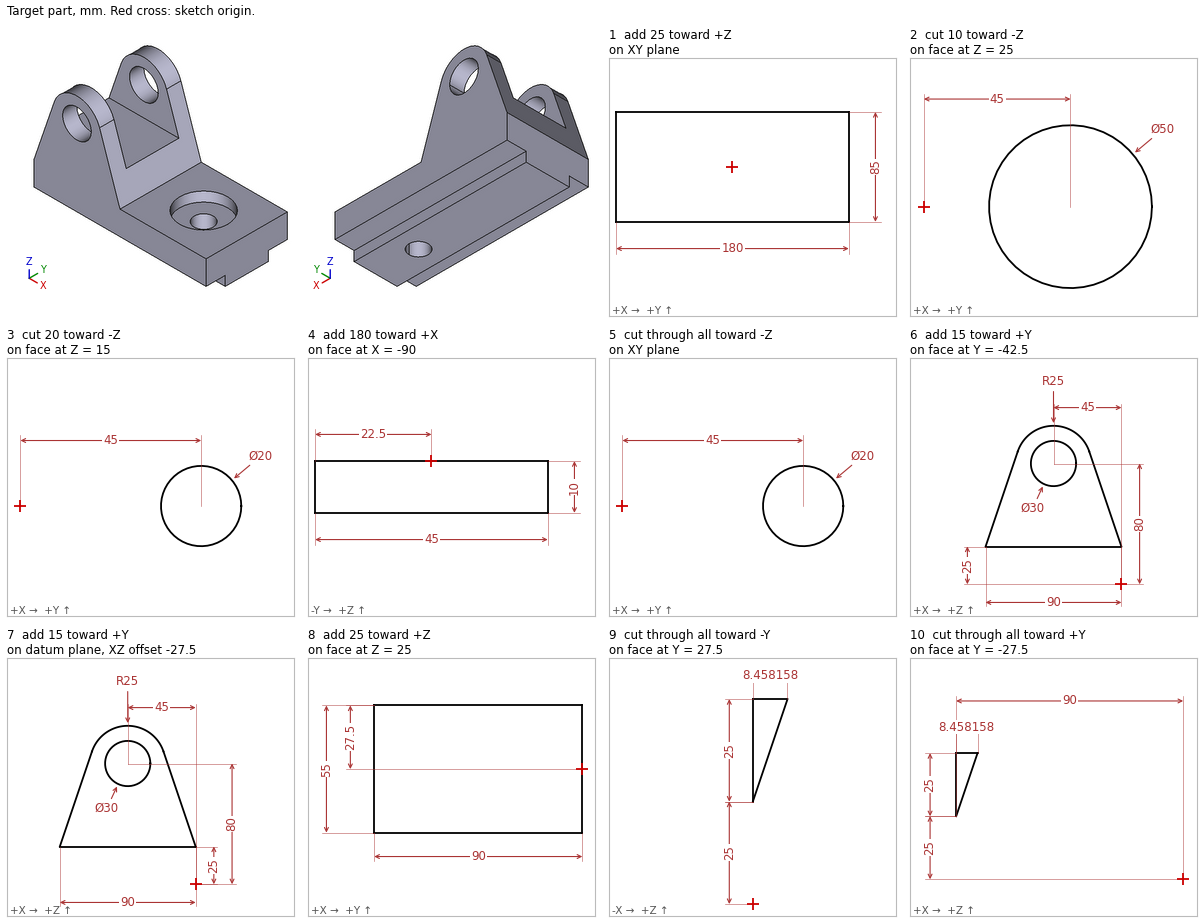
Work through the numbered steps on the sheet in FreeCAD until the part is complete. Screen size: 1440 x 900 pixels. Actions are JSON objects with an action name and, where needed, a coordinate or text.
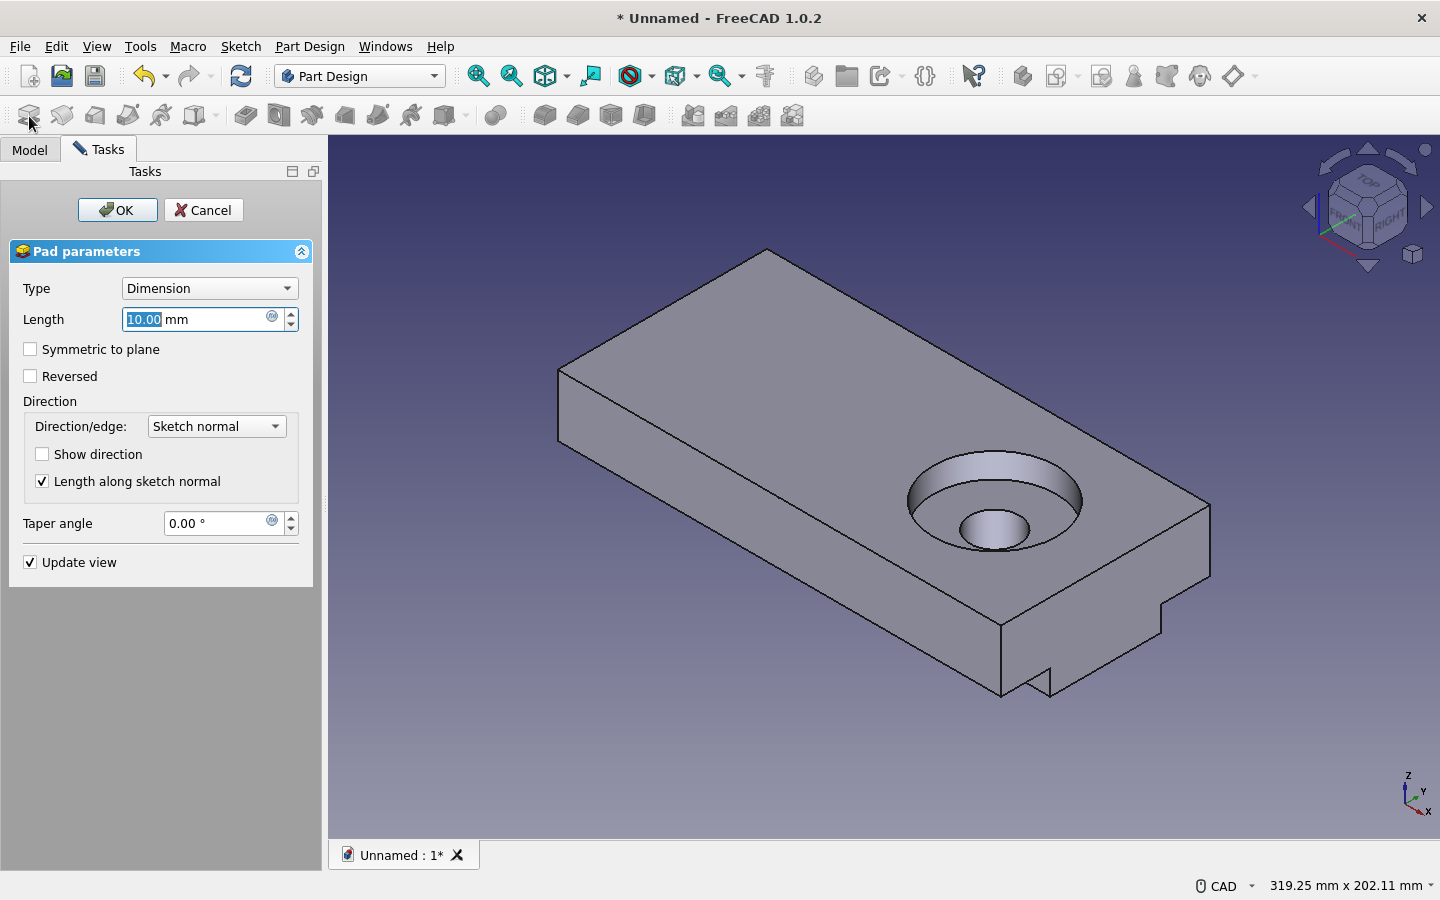
{"action": "type", "text": "15"}
{"action": "key", "text": "Tab"}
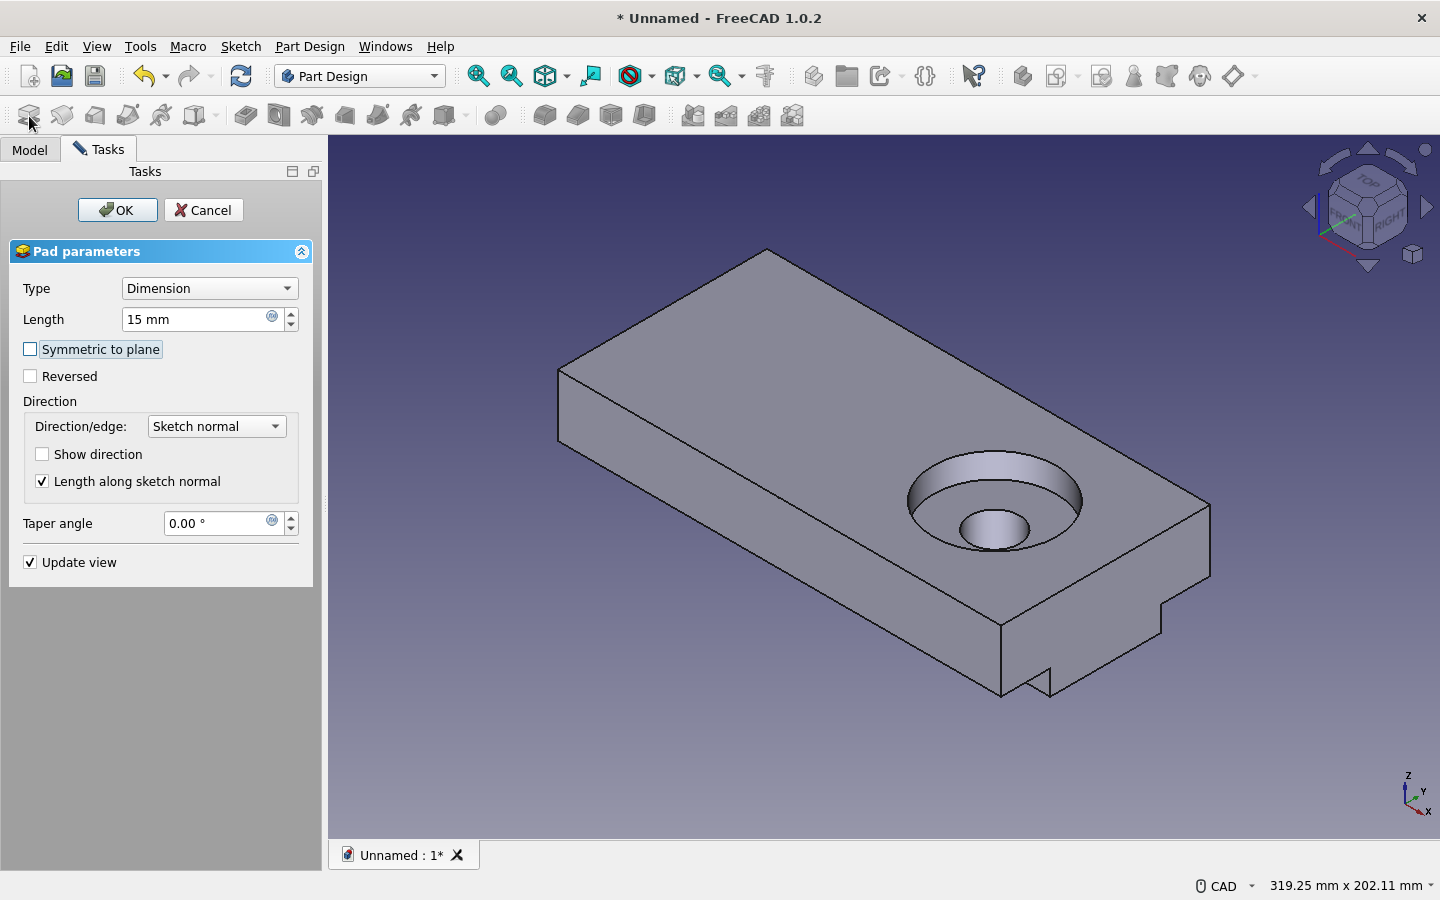
{"action": "left_click", "coordinate": [31, 376]}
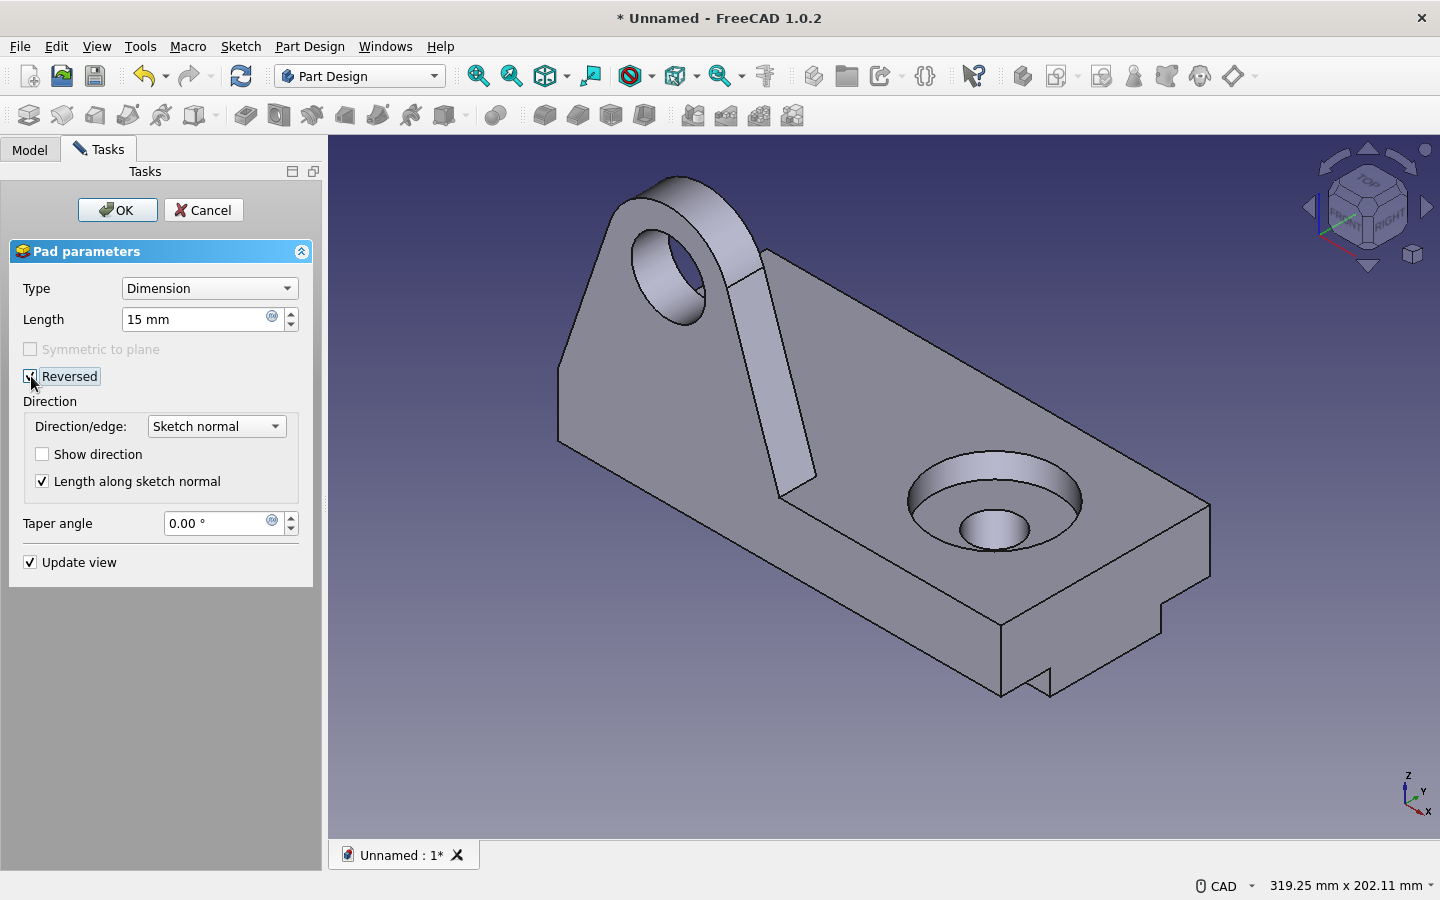
{"action": "left_click", "coordinate": [118, 210]}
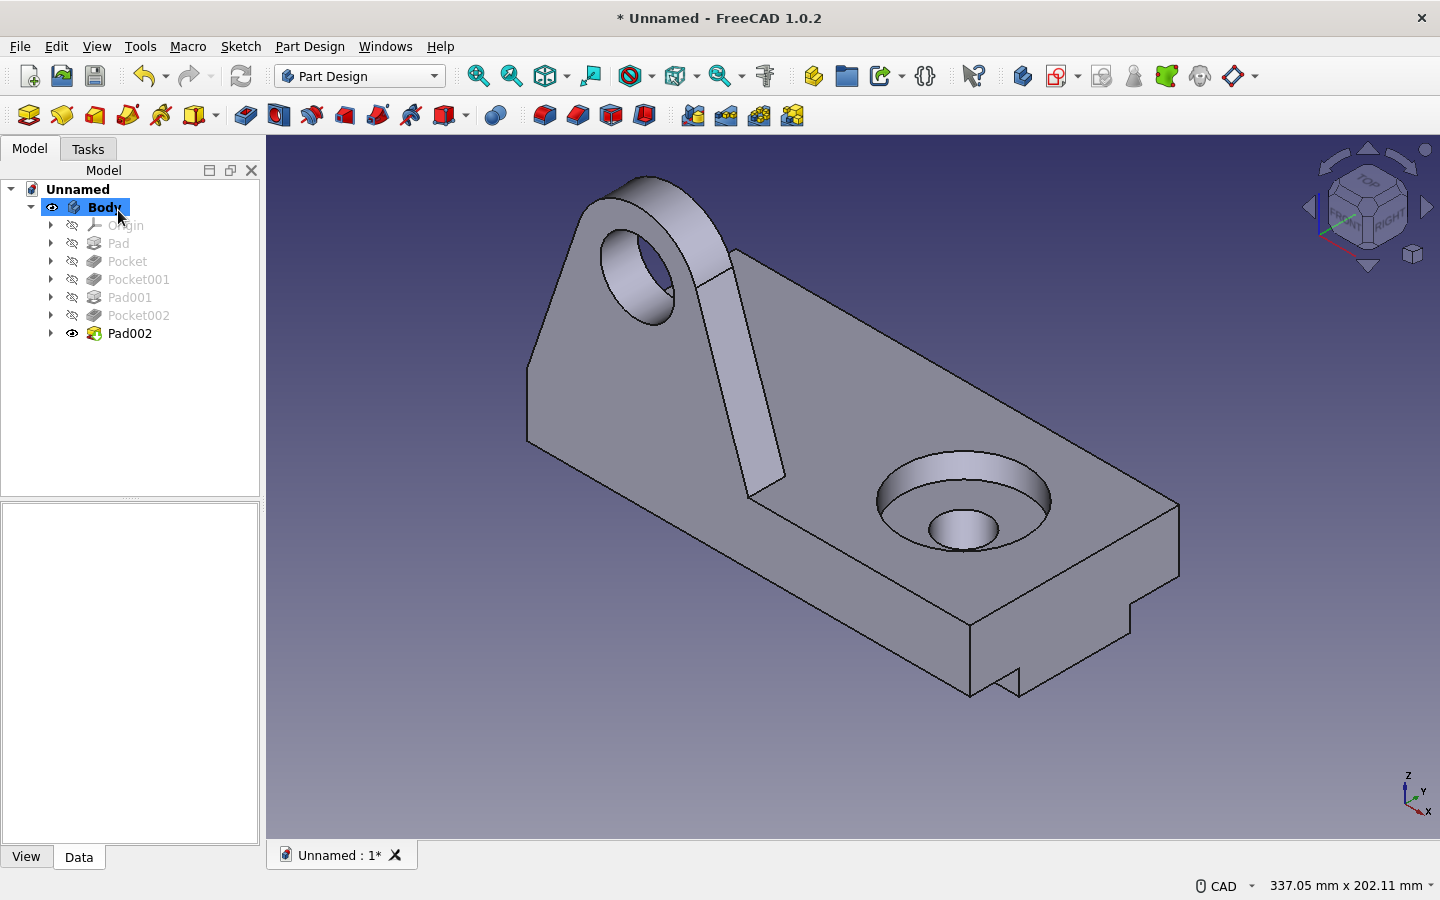
{"action": "left_click", "coordinate": [479, 76]}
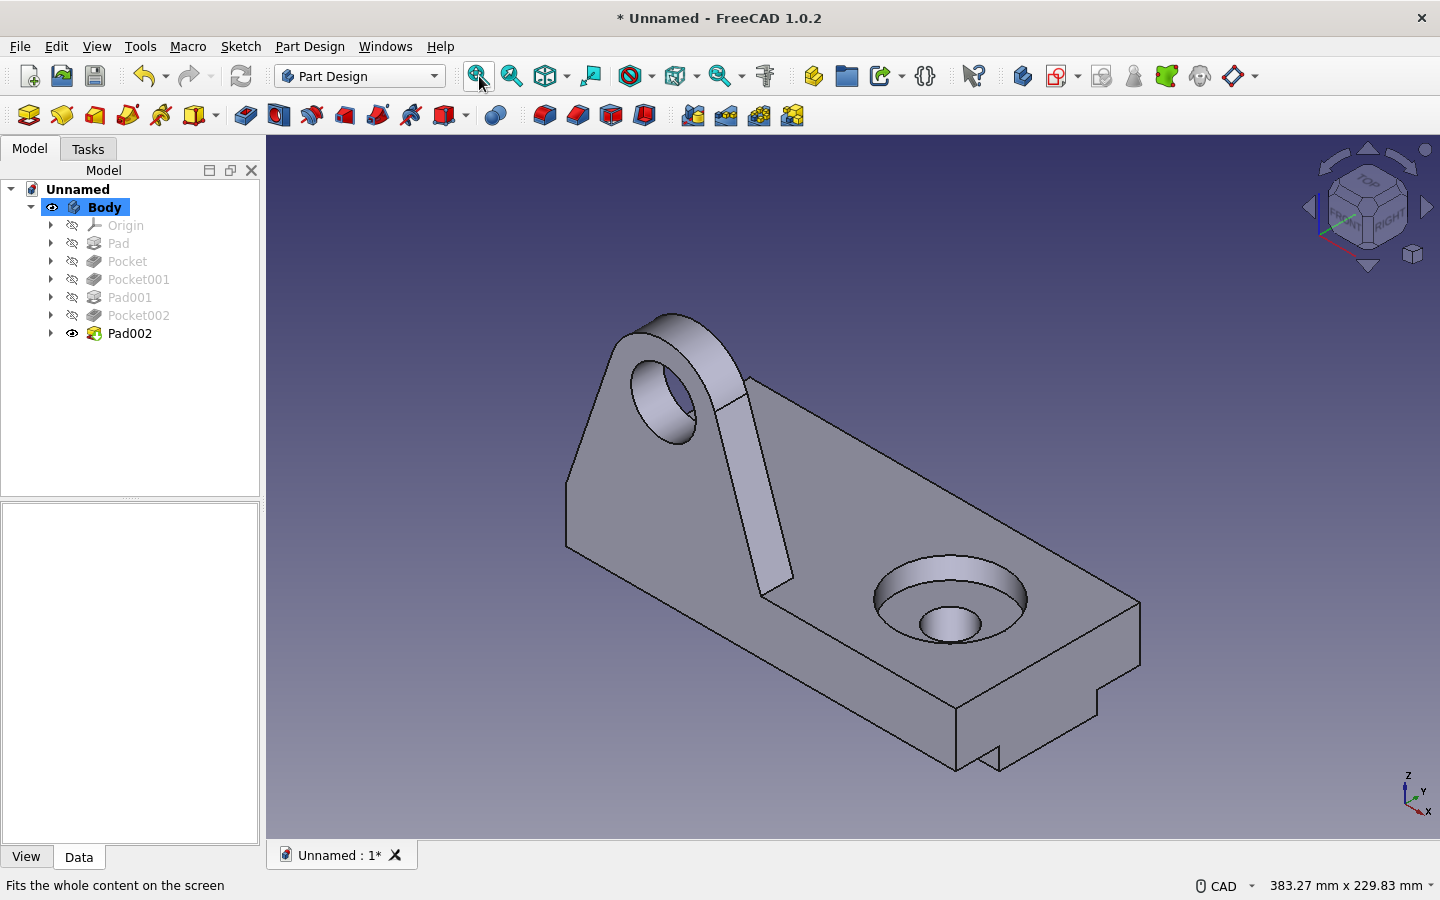
{"action": "left_click", "coordinate": [51, 225]}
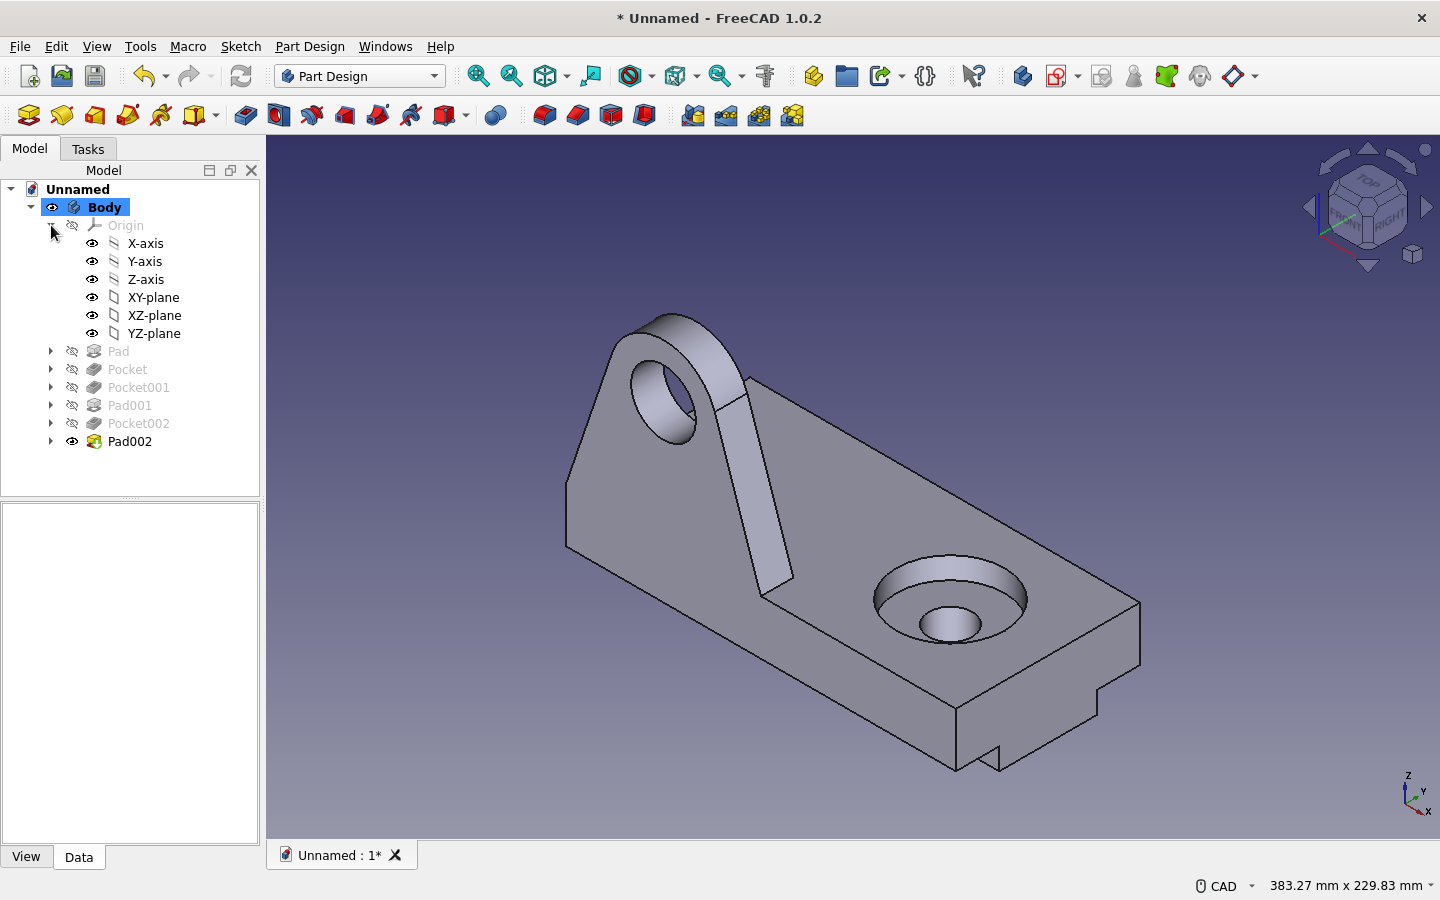
{"action": "left_click", "coordinate": [137, 315]}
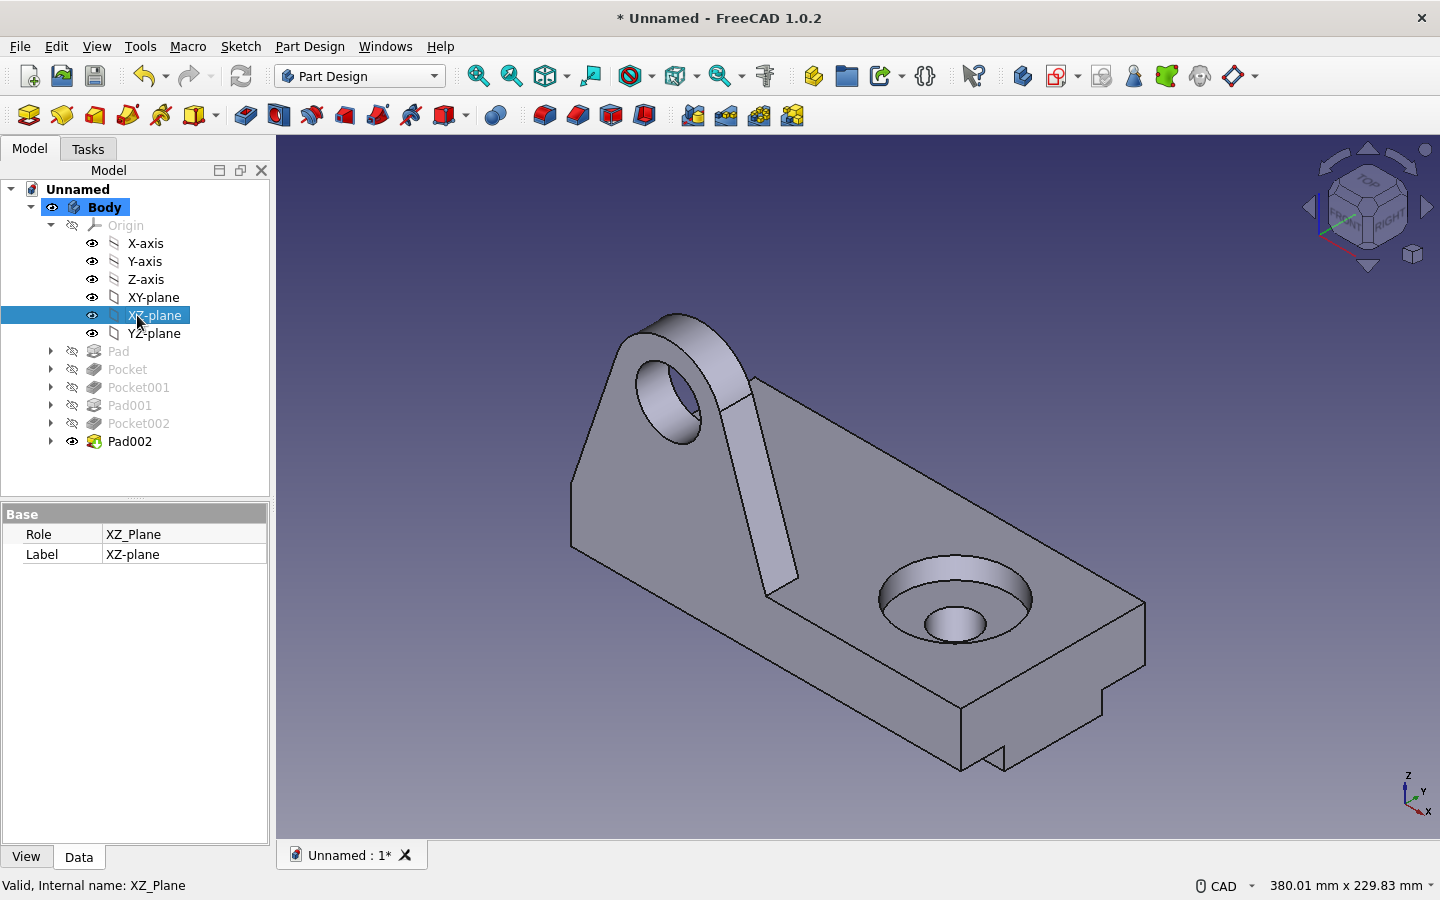
{"action": "left_click", "coordinate": [1232, 76]}